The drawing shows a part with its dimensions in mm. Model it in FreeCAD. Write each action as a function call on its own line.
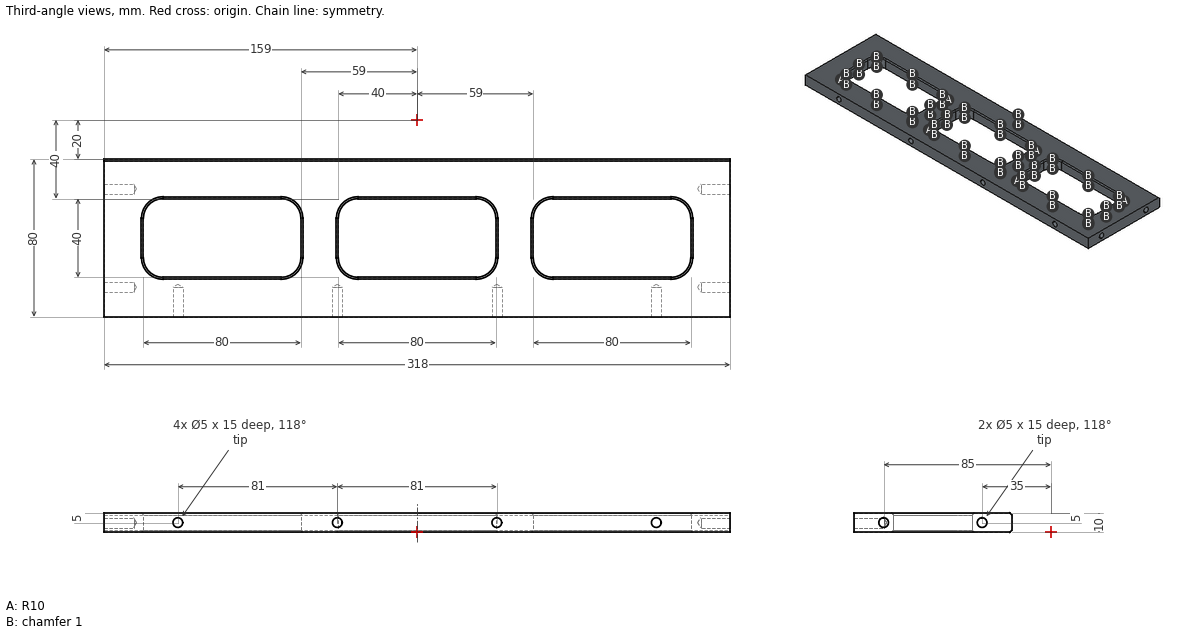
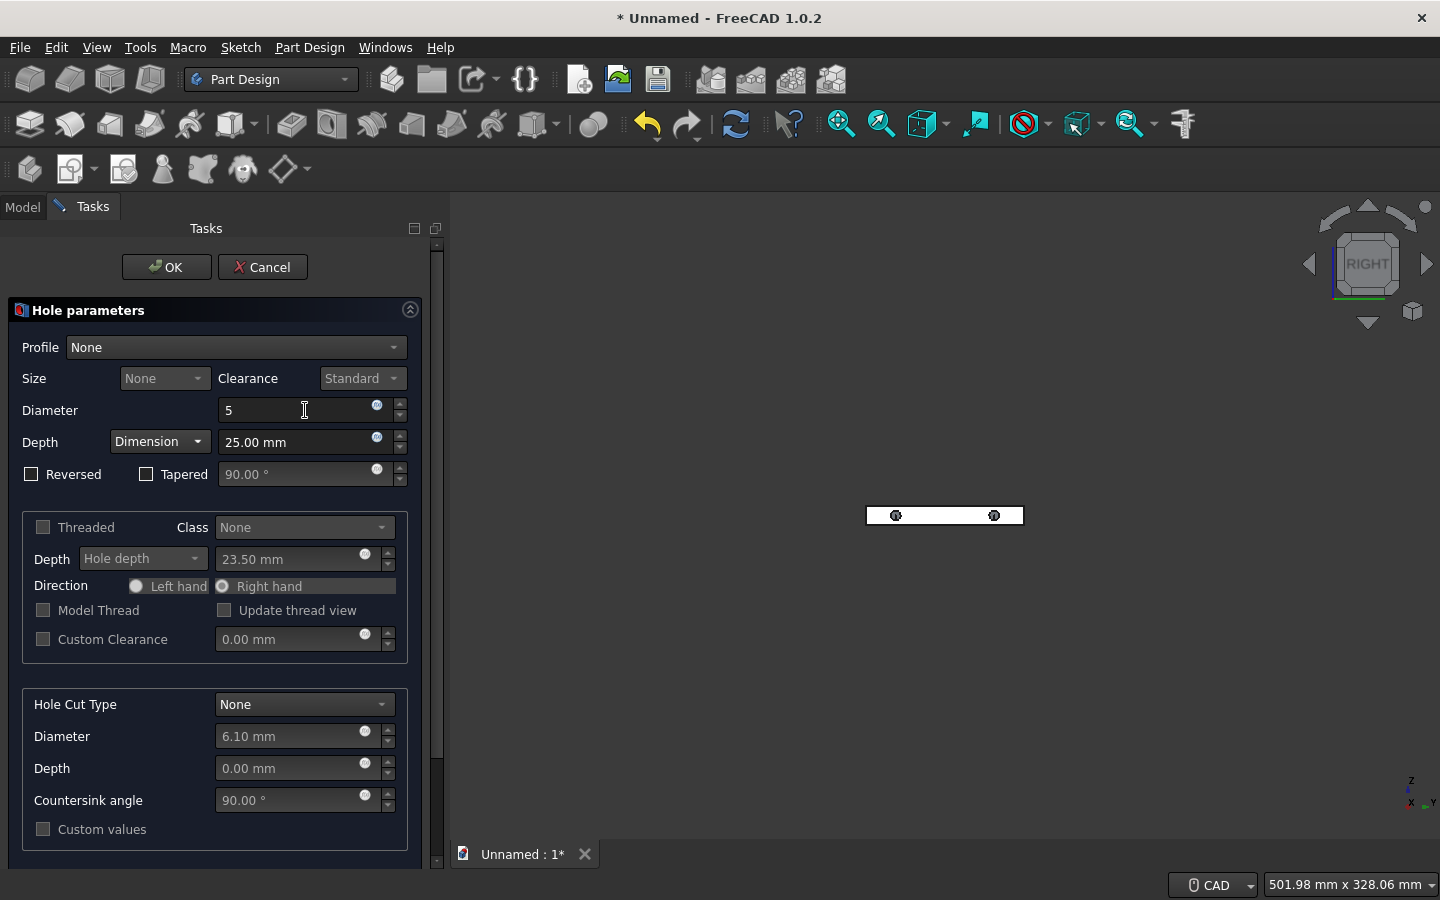
triple_click(305, 442)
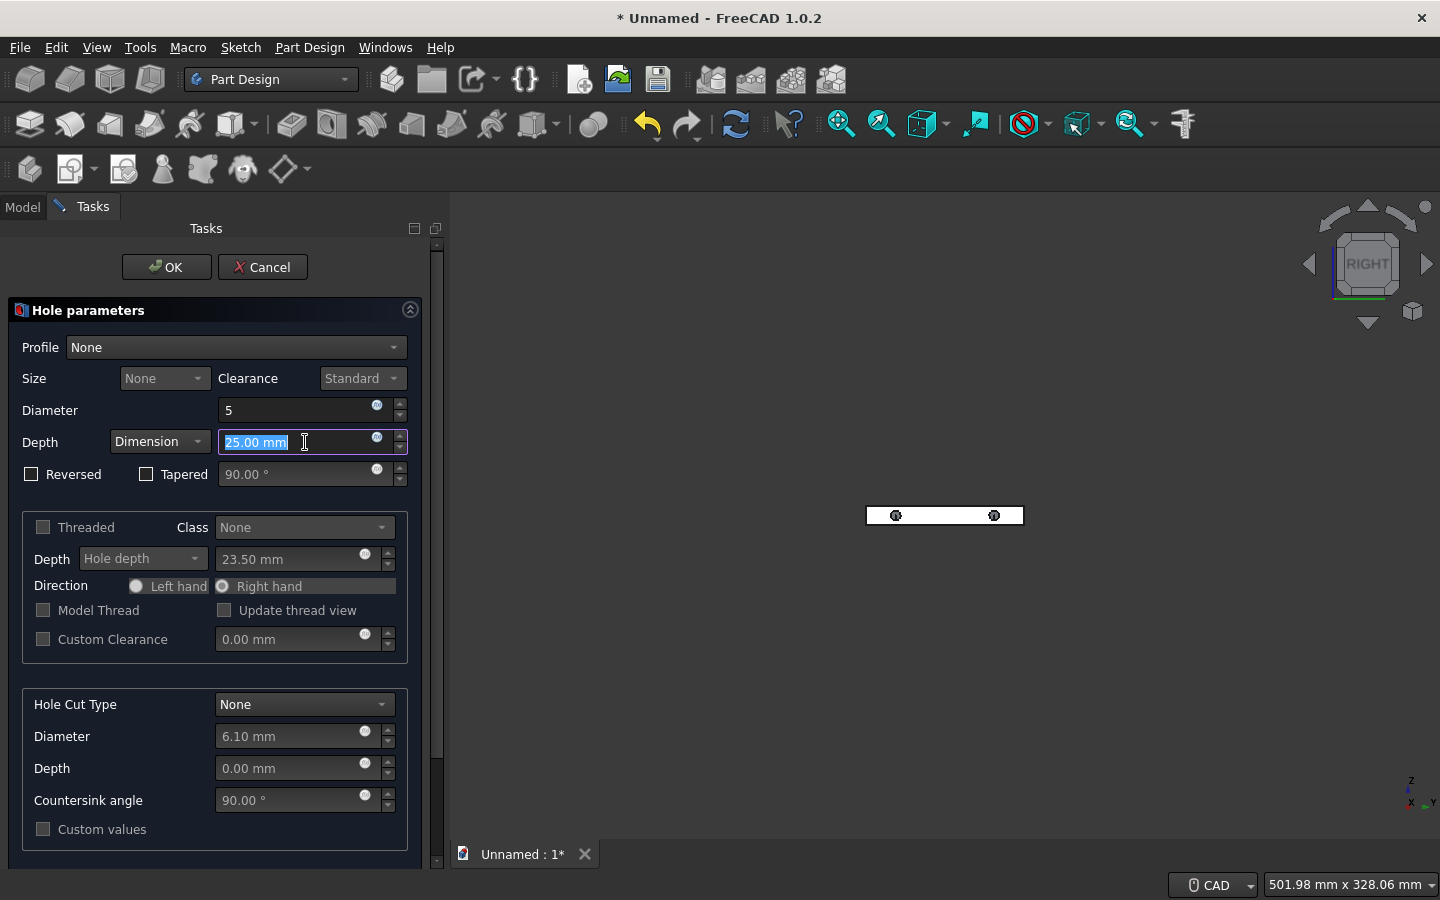
text(15)
key(Tab)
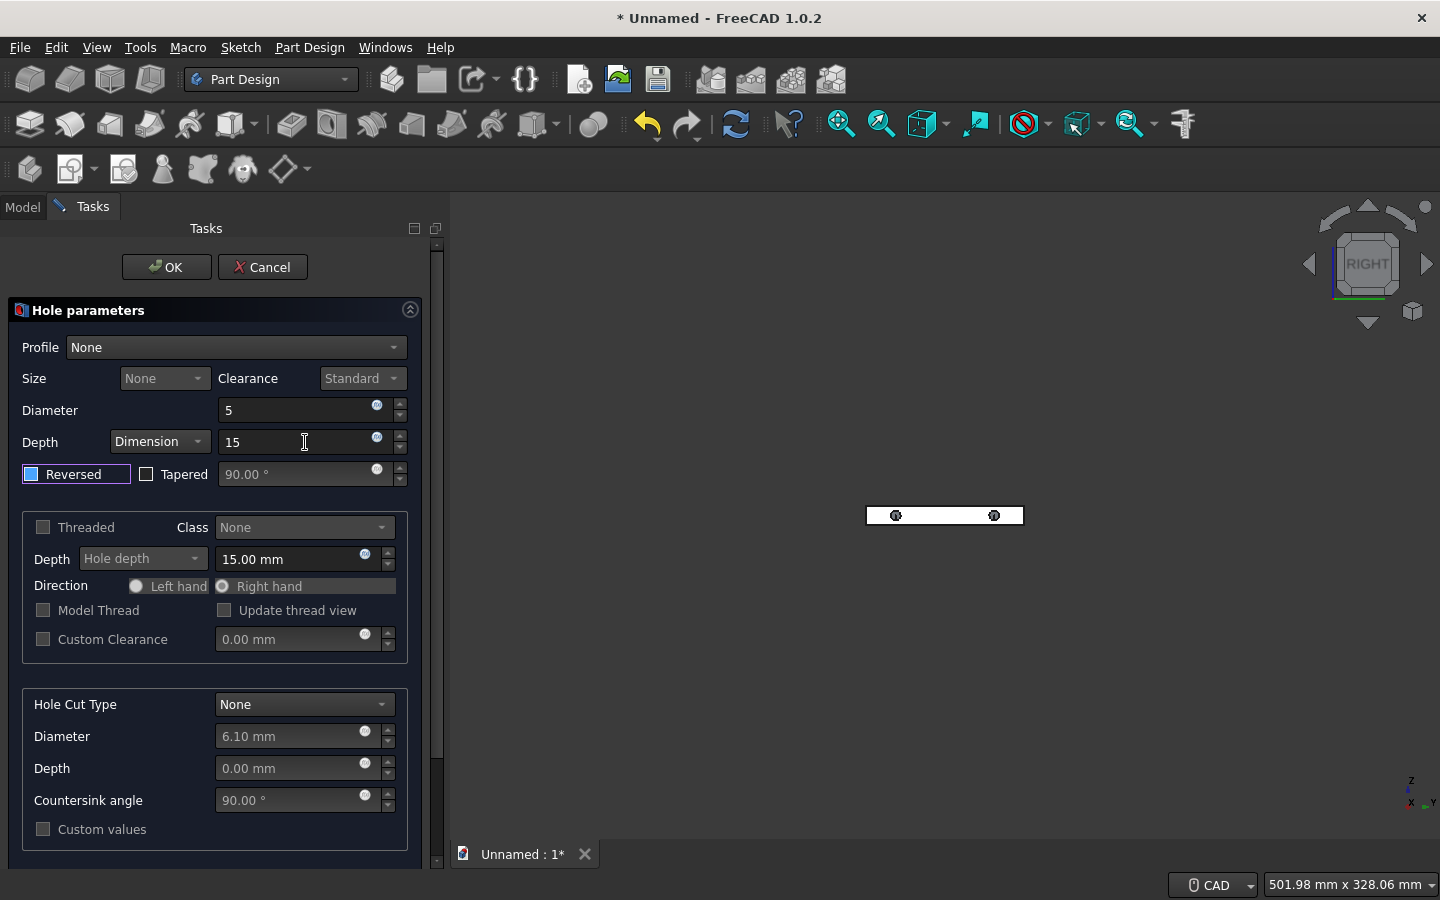
click(167, 267)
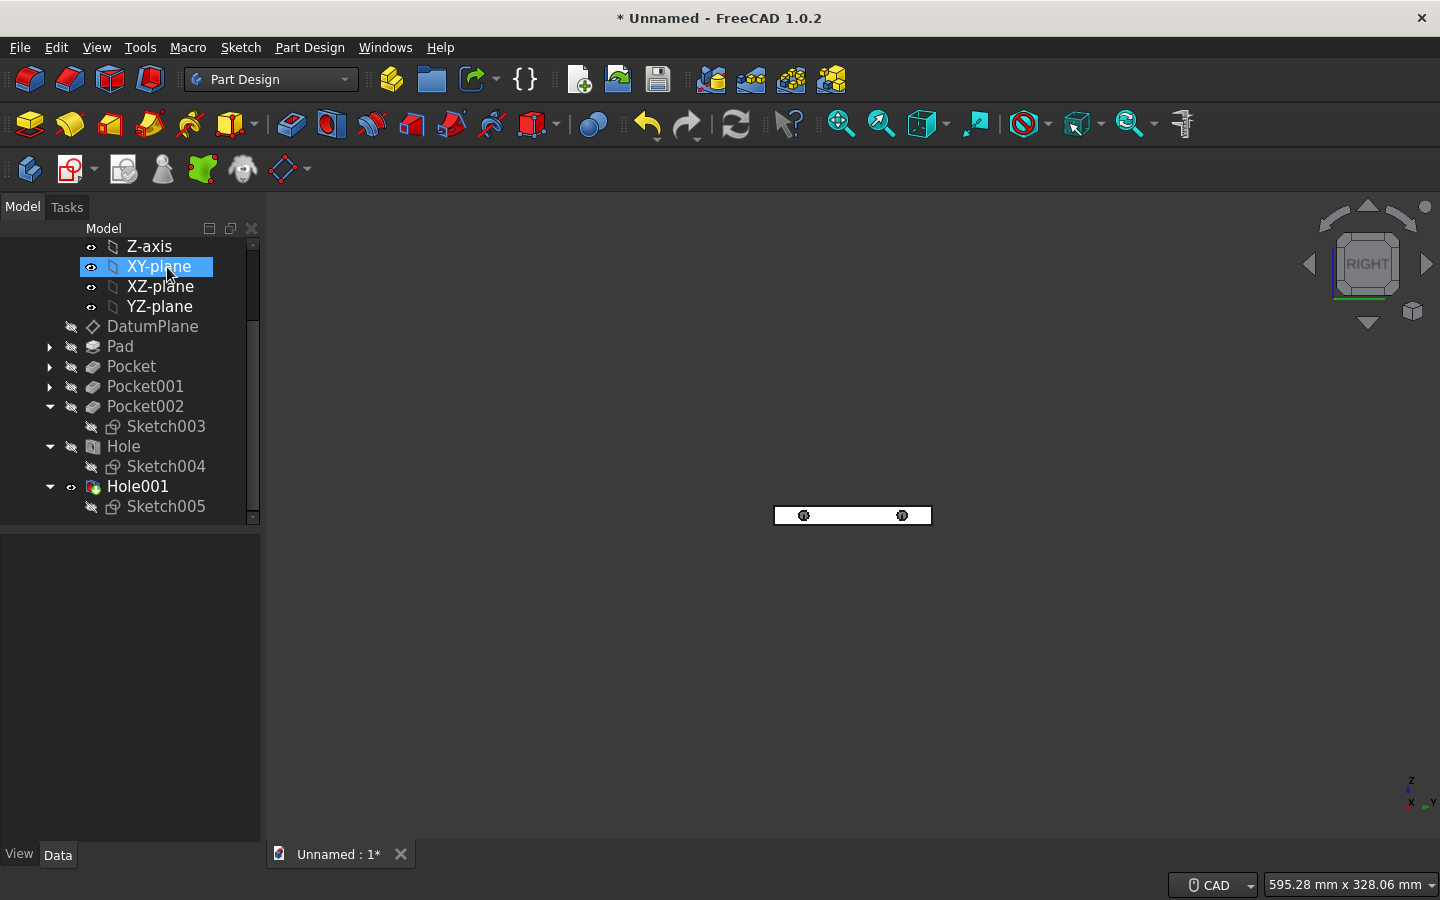
click(842, 124)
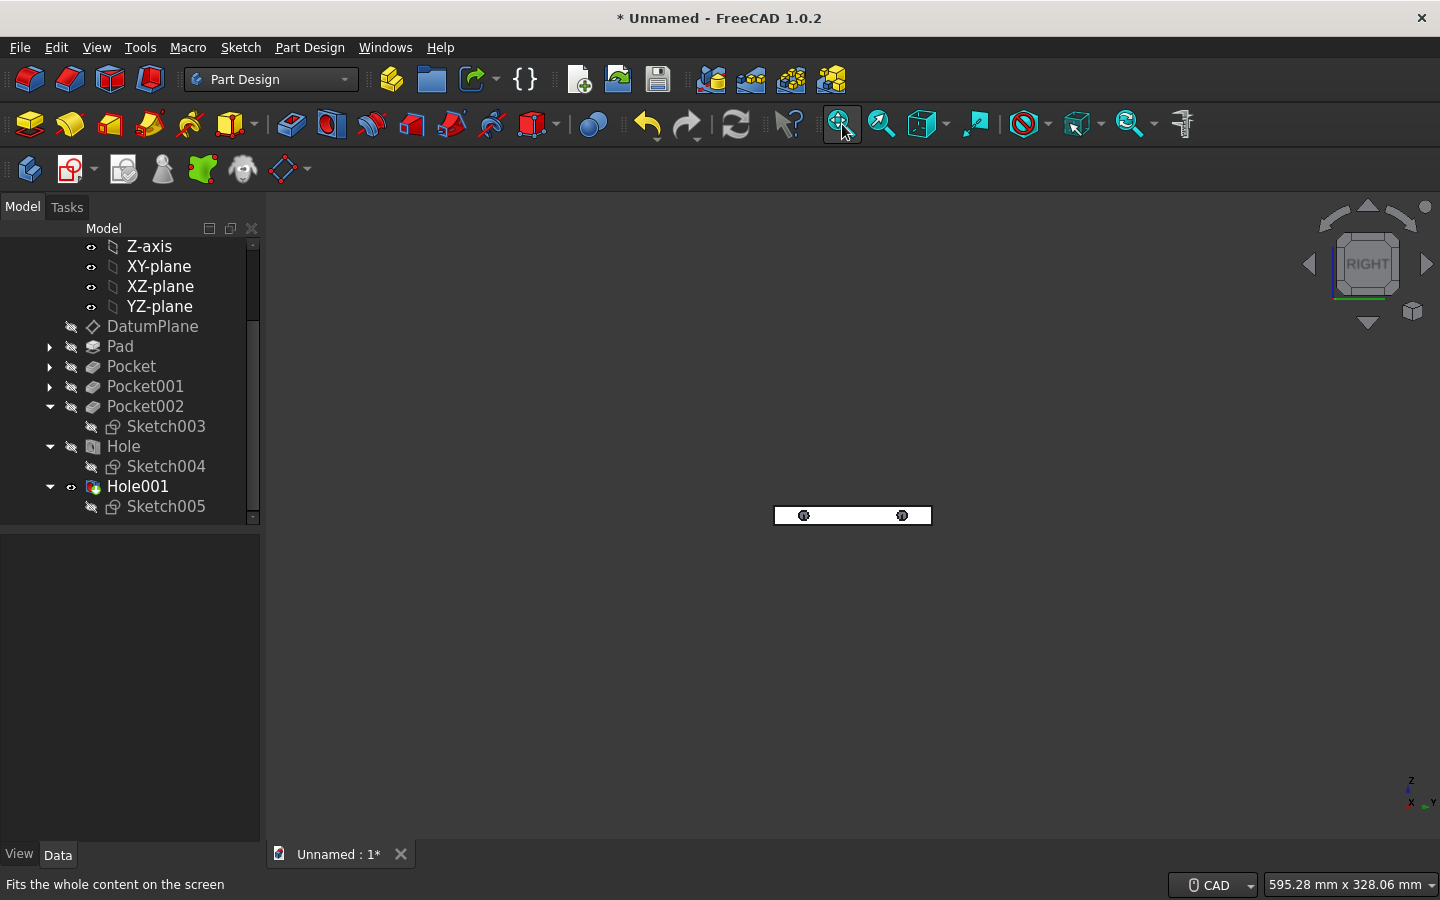
key(0)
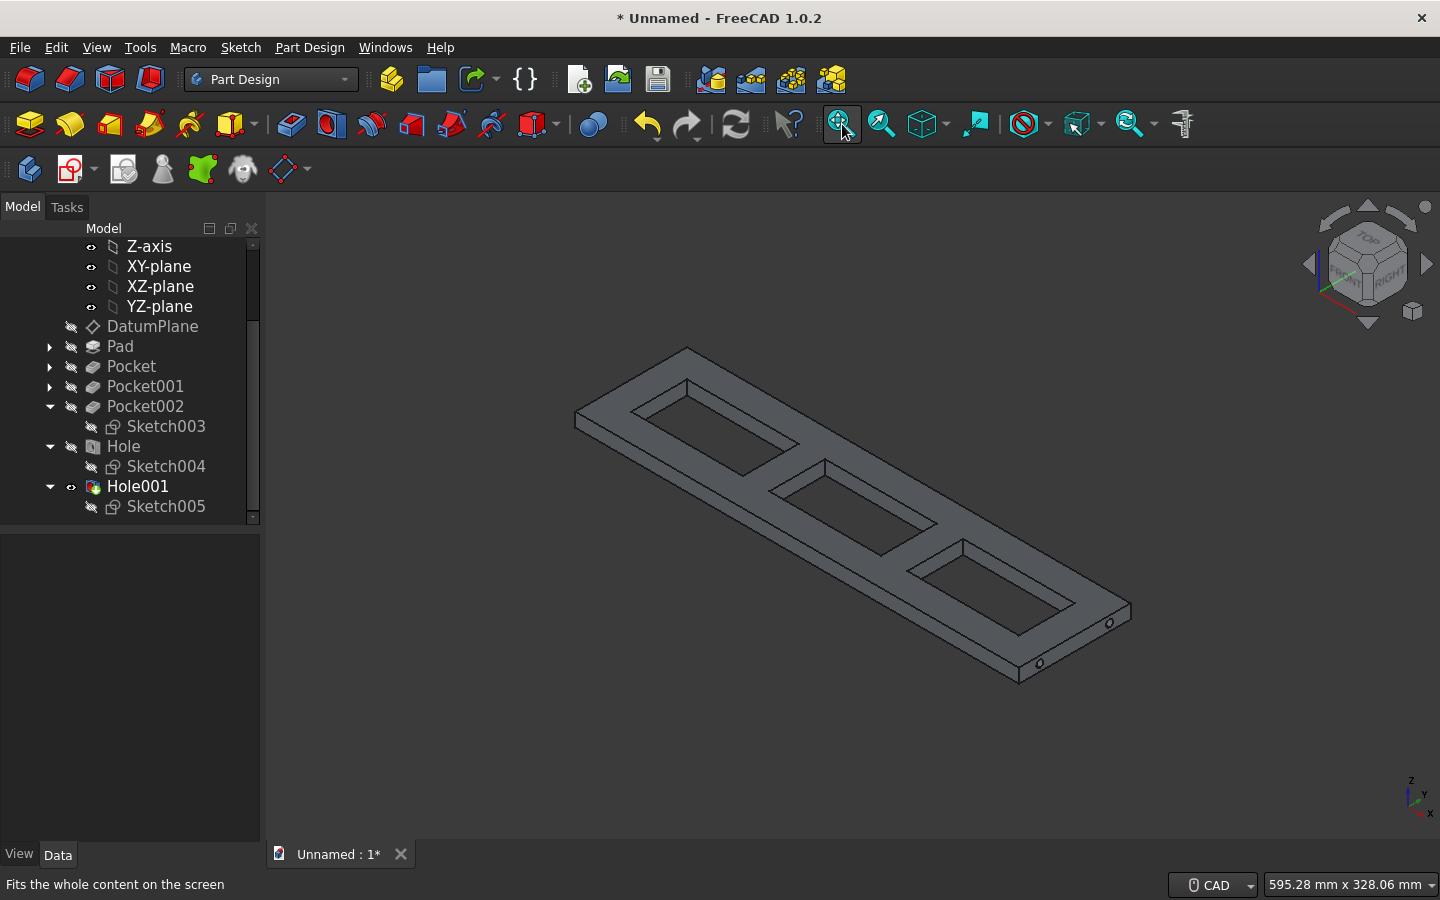
key(1)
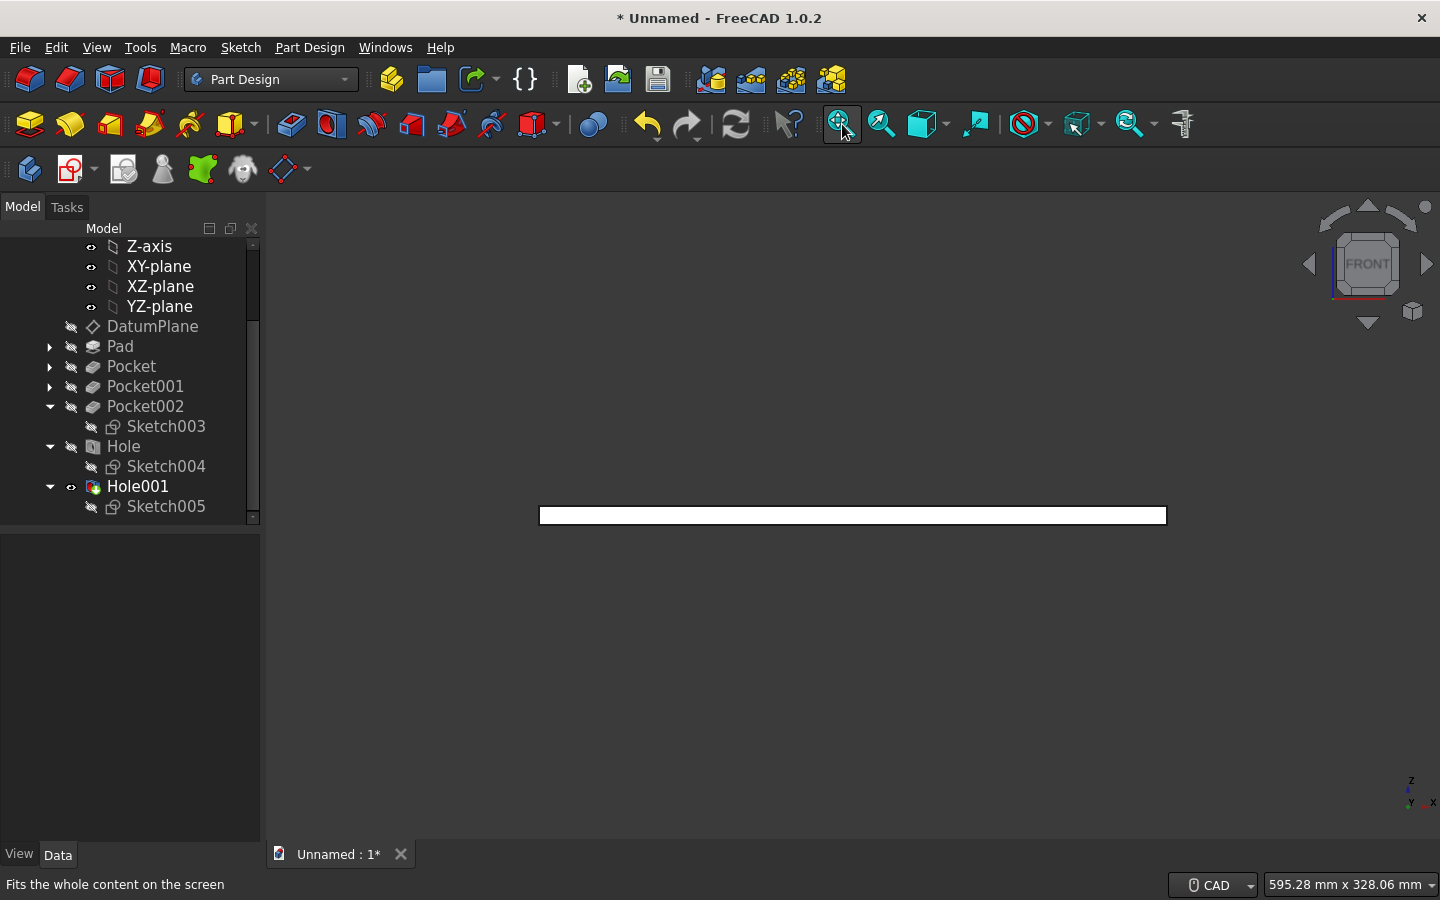
click(1122, 514)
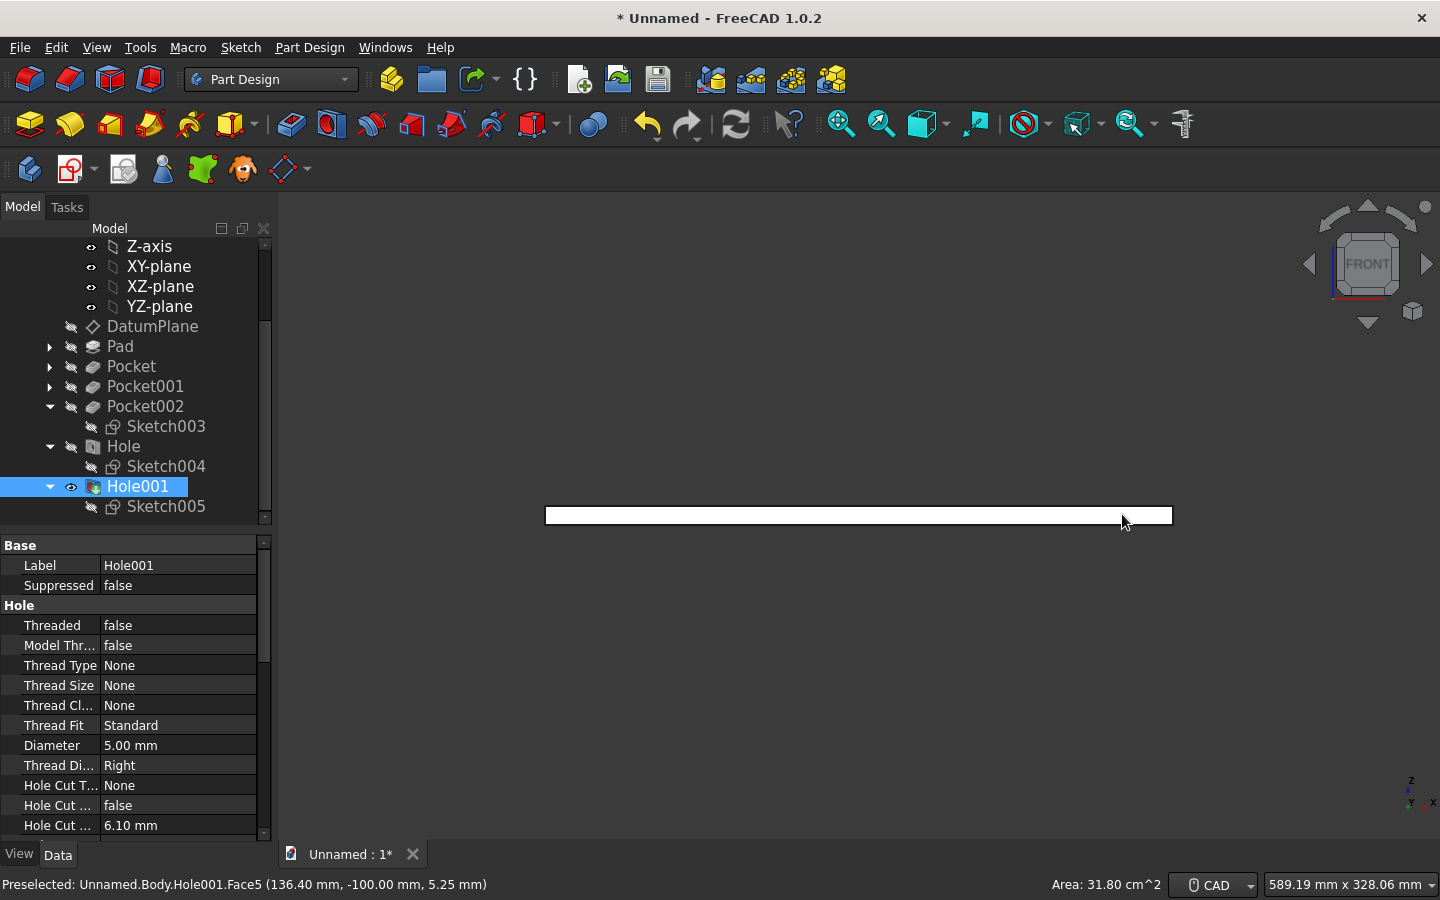
click(70, 170)